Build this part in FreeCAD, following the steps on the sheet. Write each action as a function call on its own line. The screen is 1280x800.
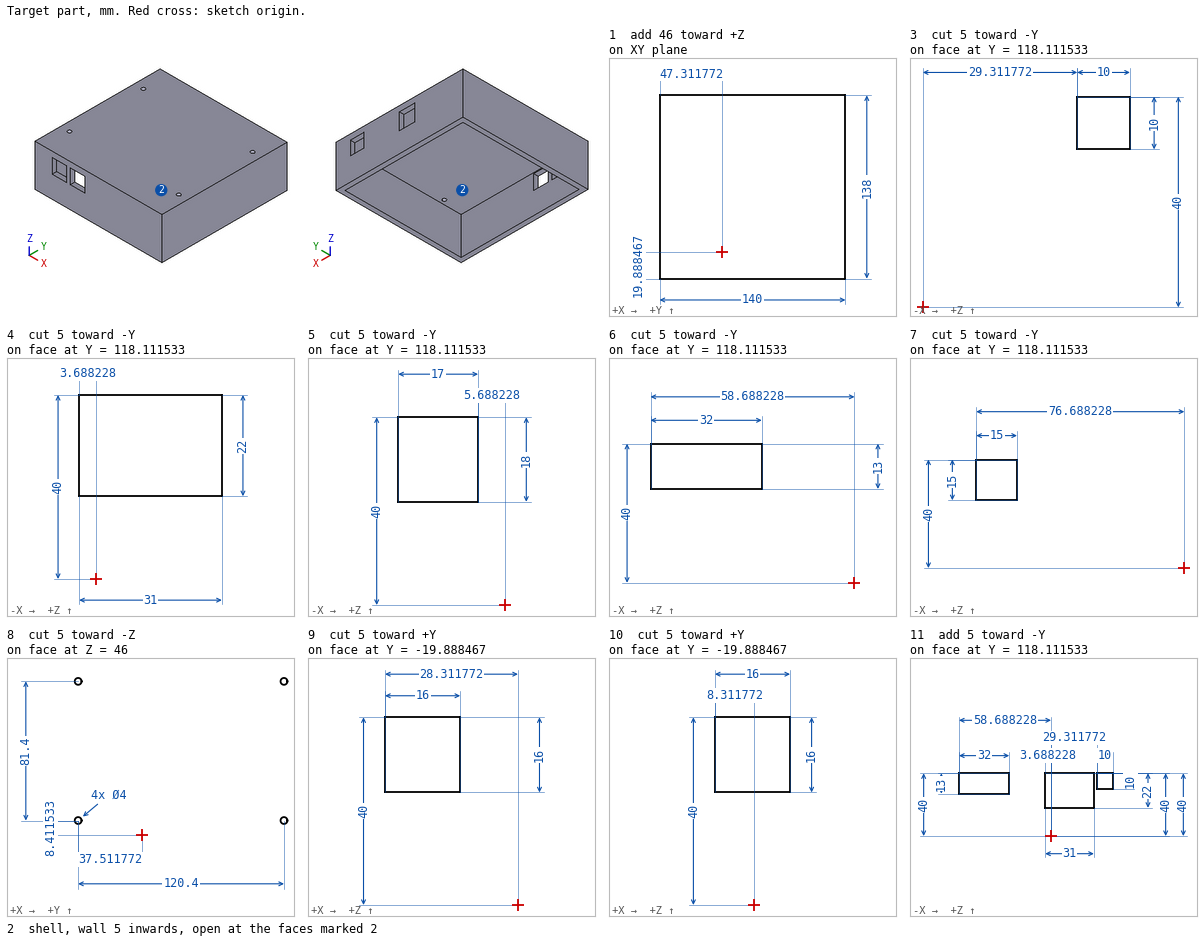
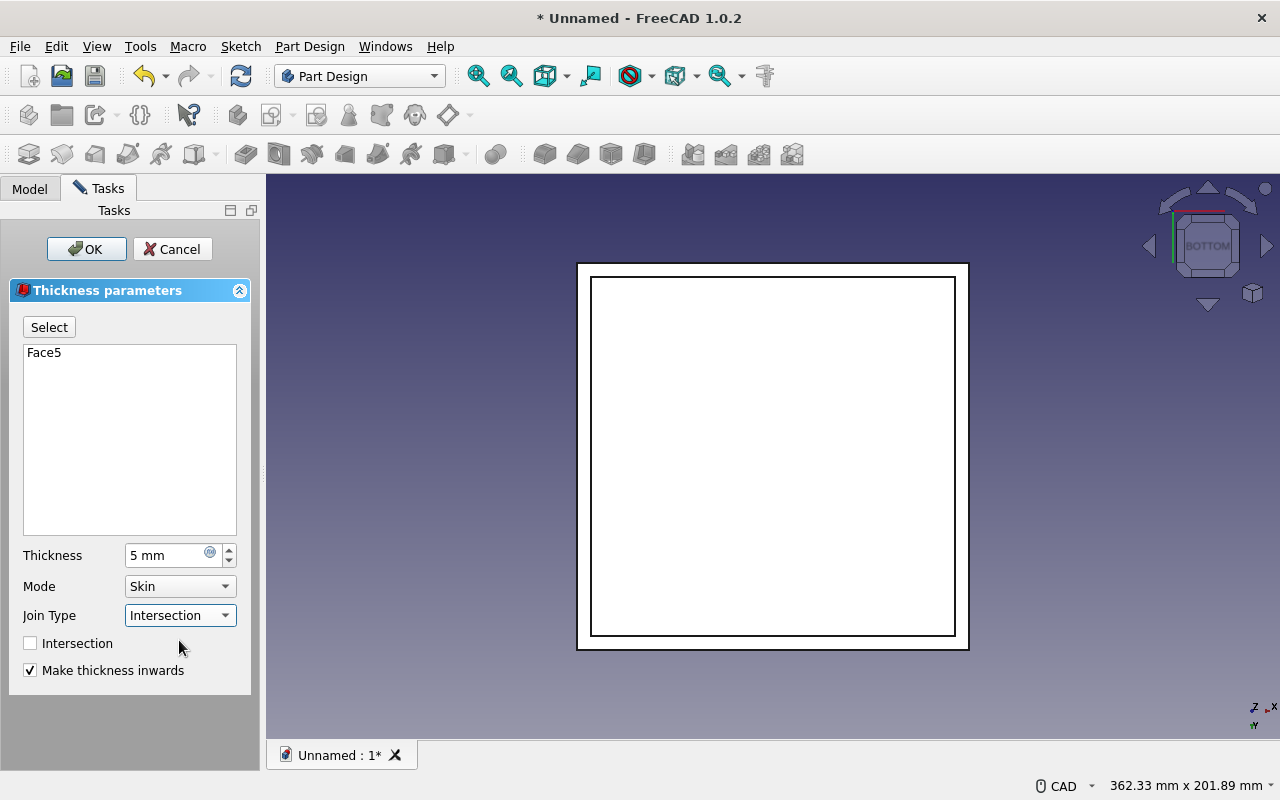
click(87, 249)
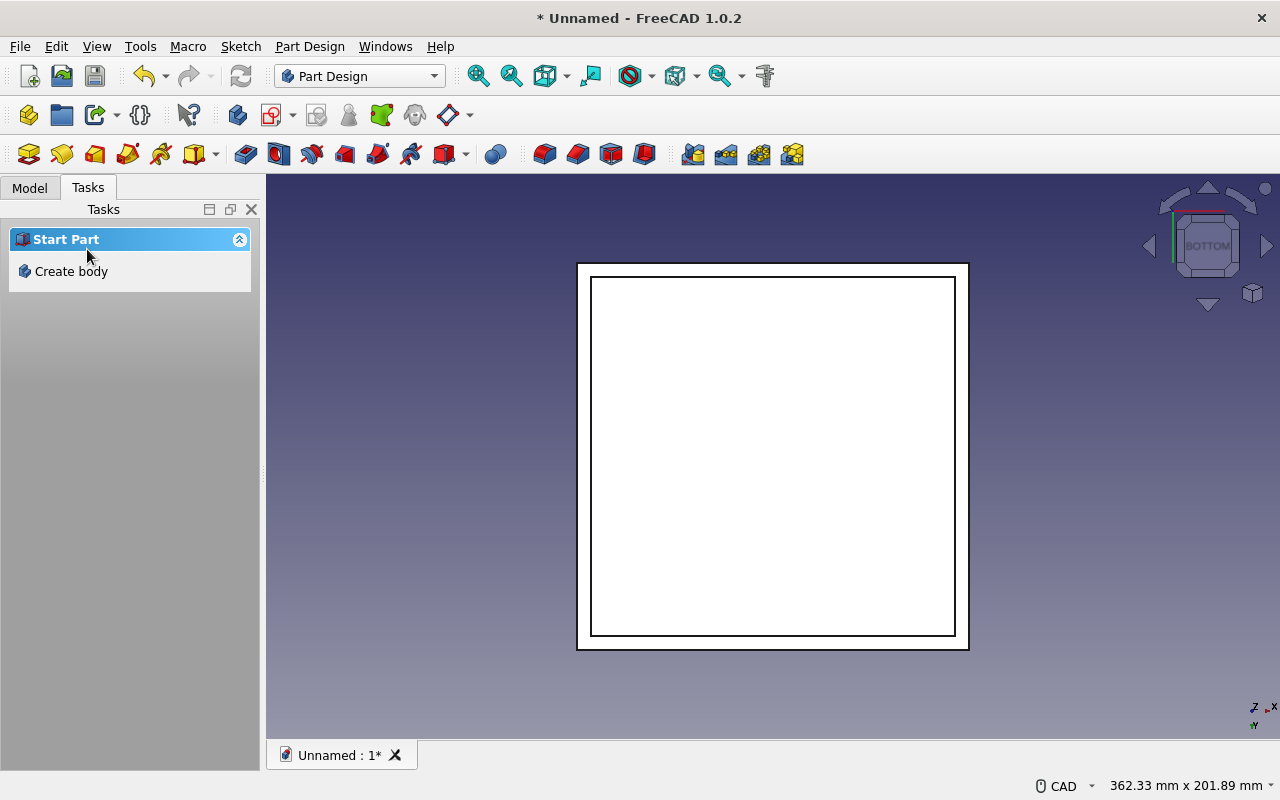
key(4)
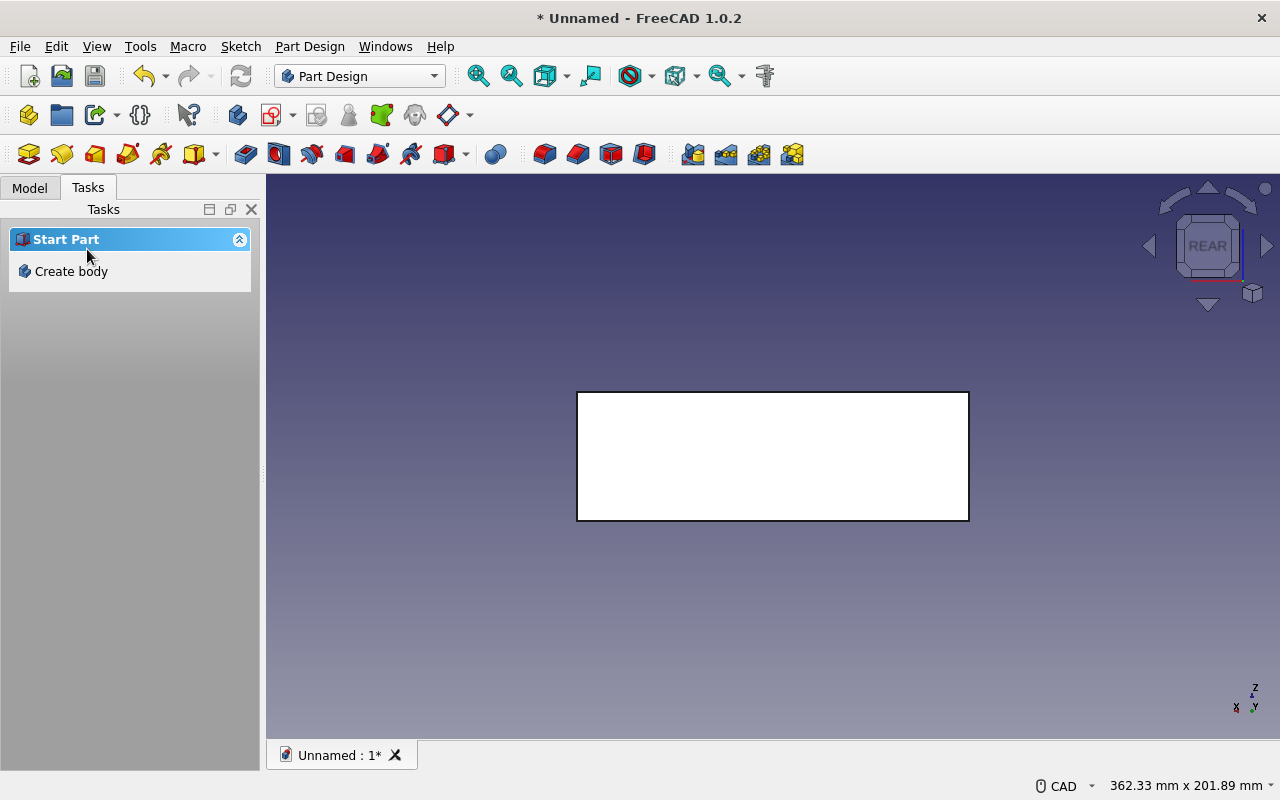
click(479, 76)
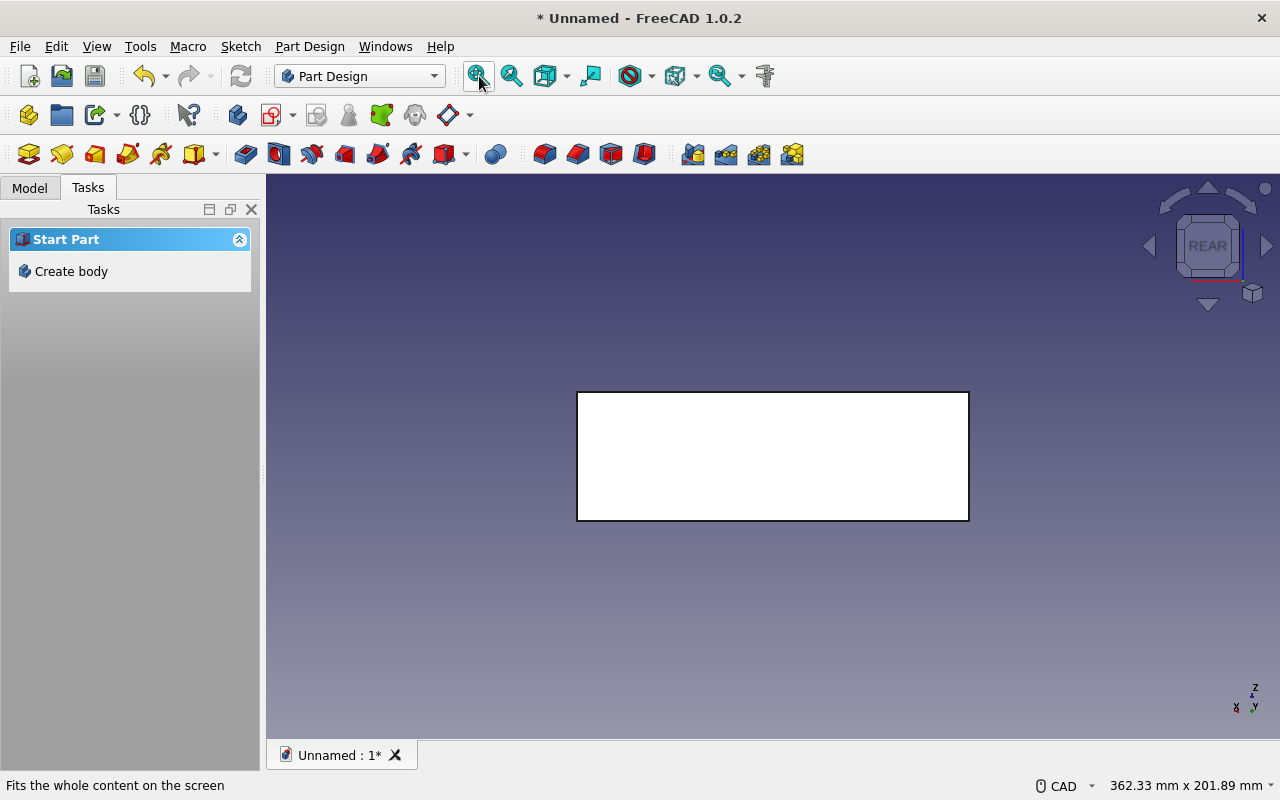
click(661, 456)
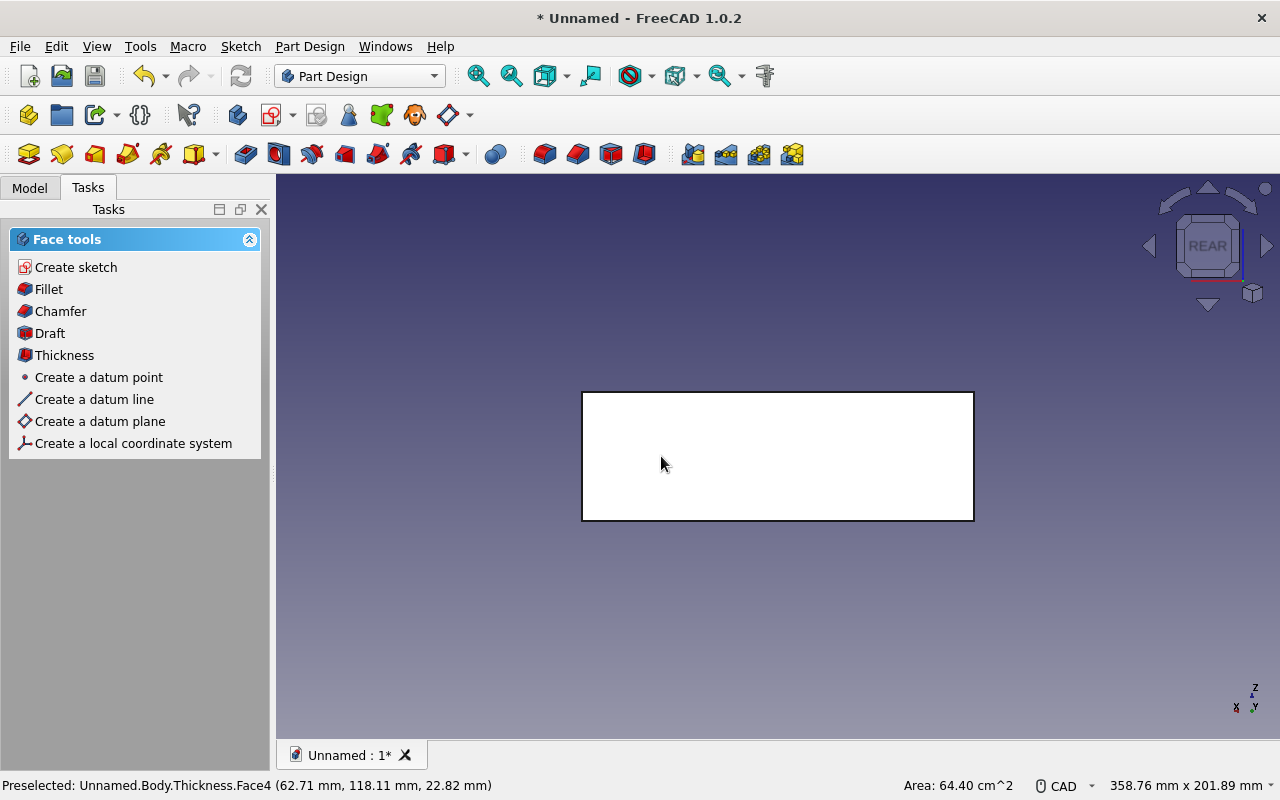
click(270, 116)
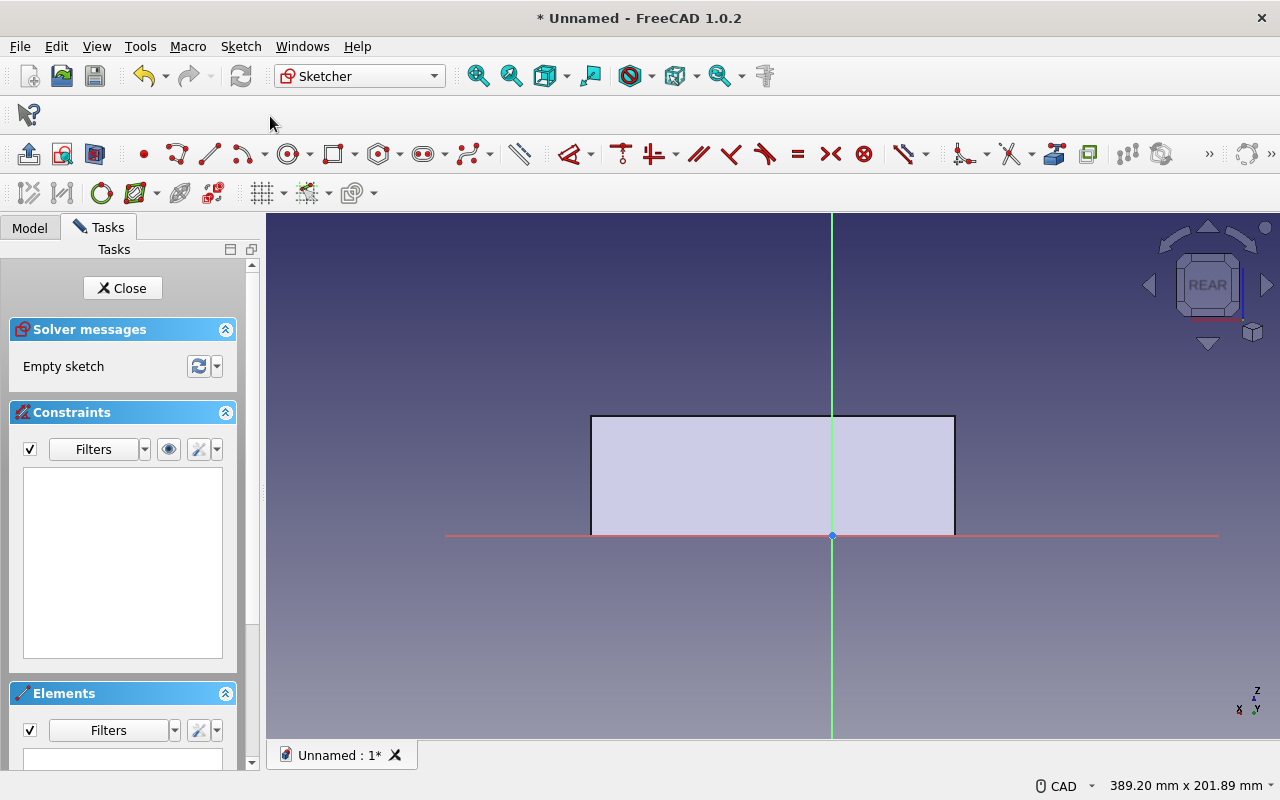
scroll(939, 442, up, 13)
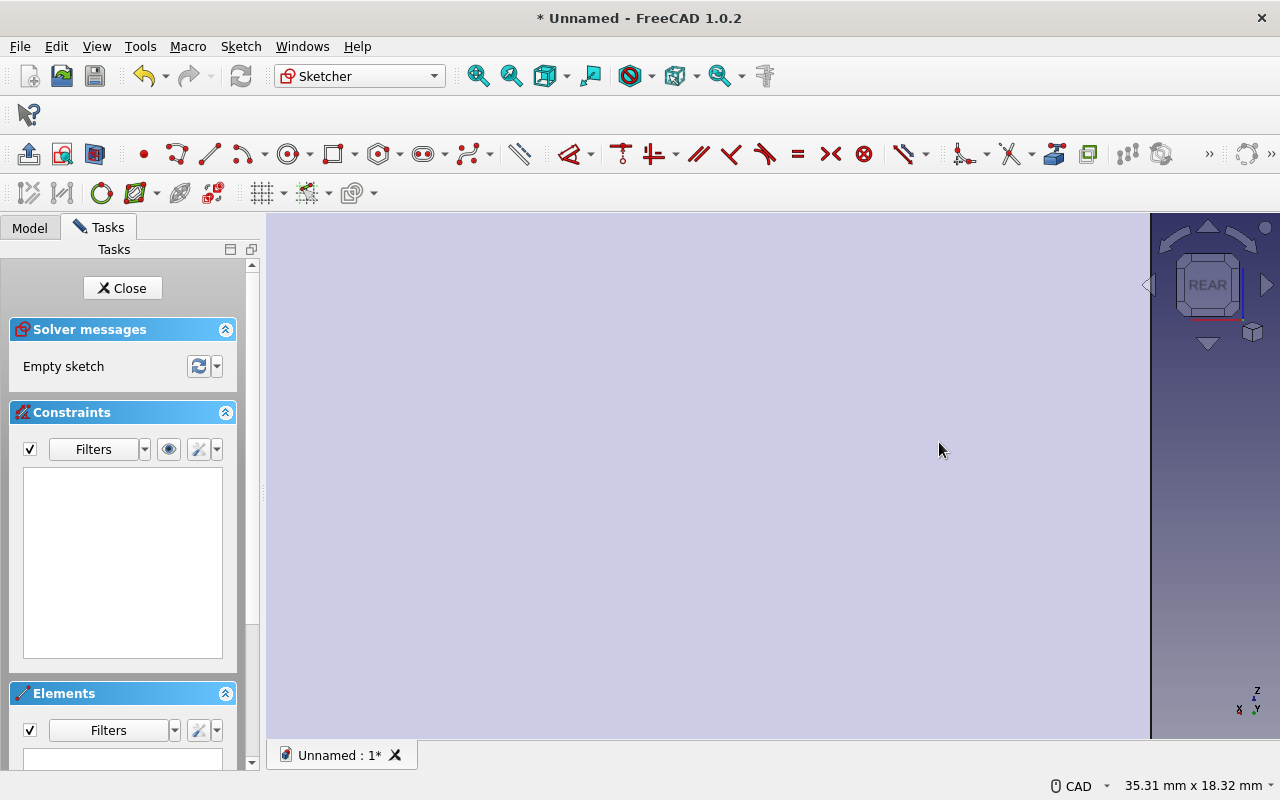
key(g)
key(r)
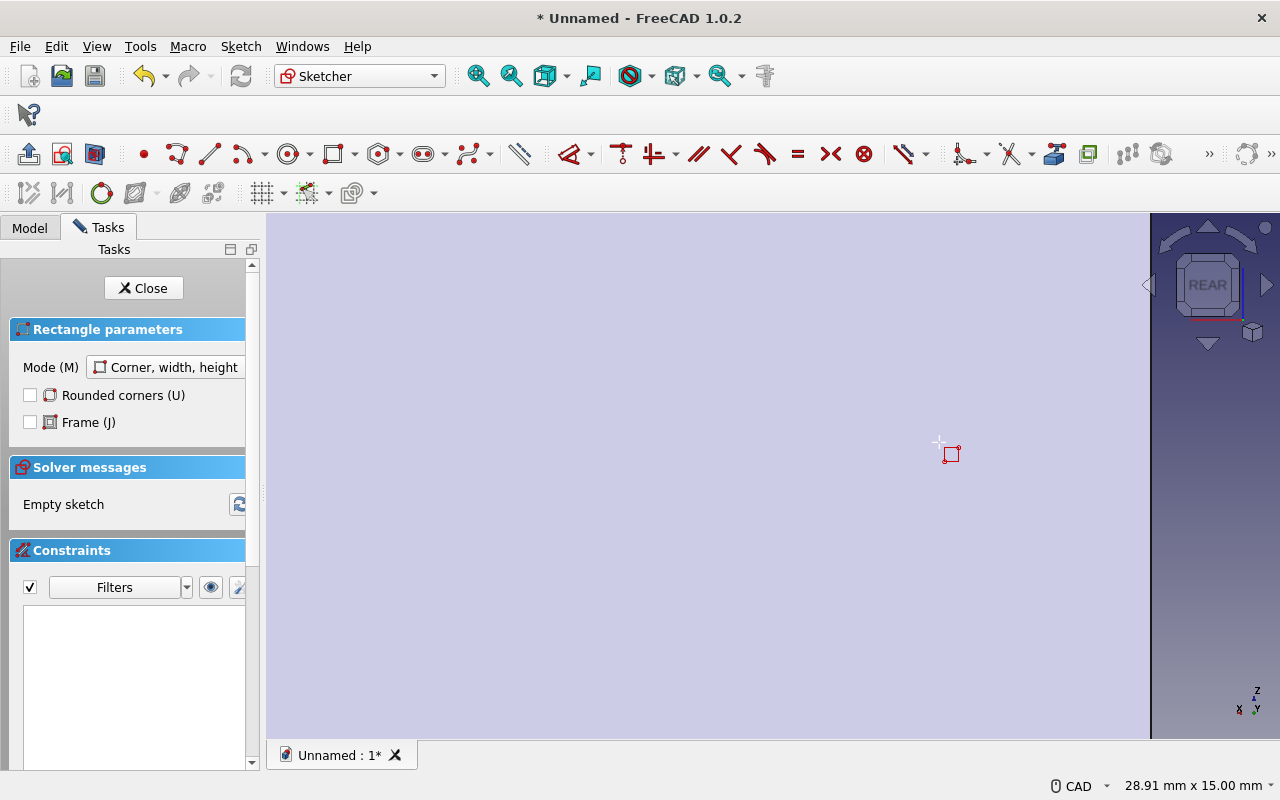
click(520, 298)
move(871, 649)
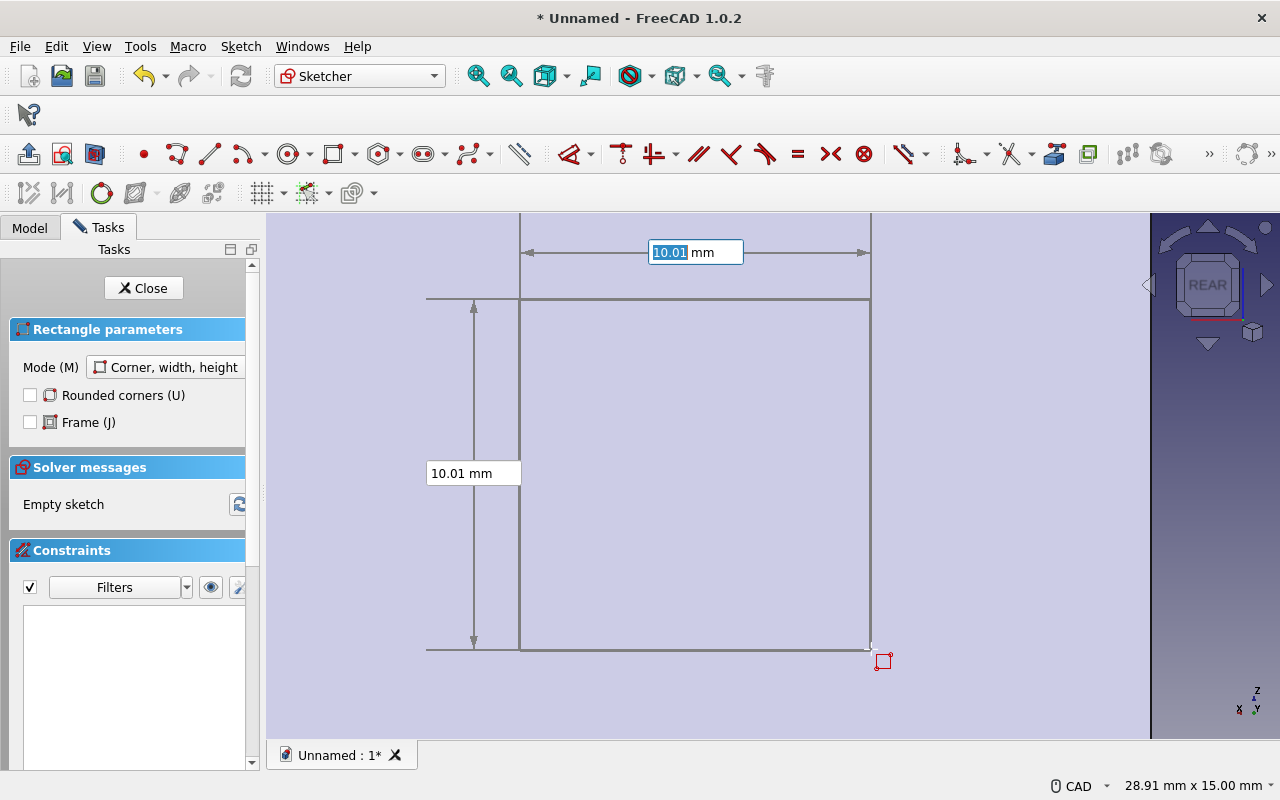
text(10)
key(Tab)
text(10)
key(Return)
key(Escape)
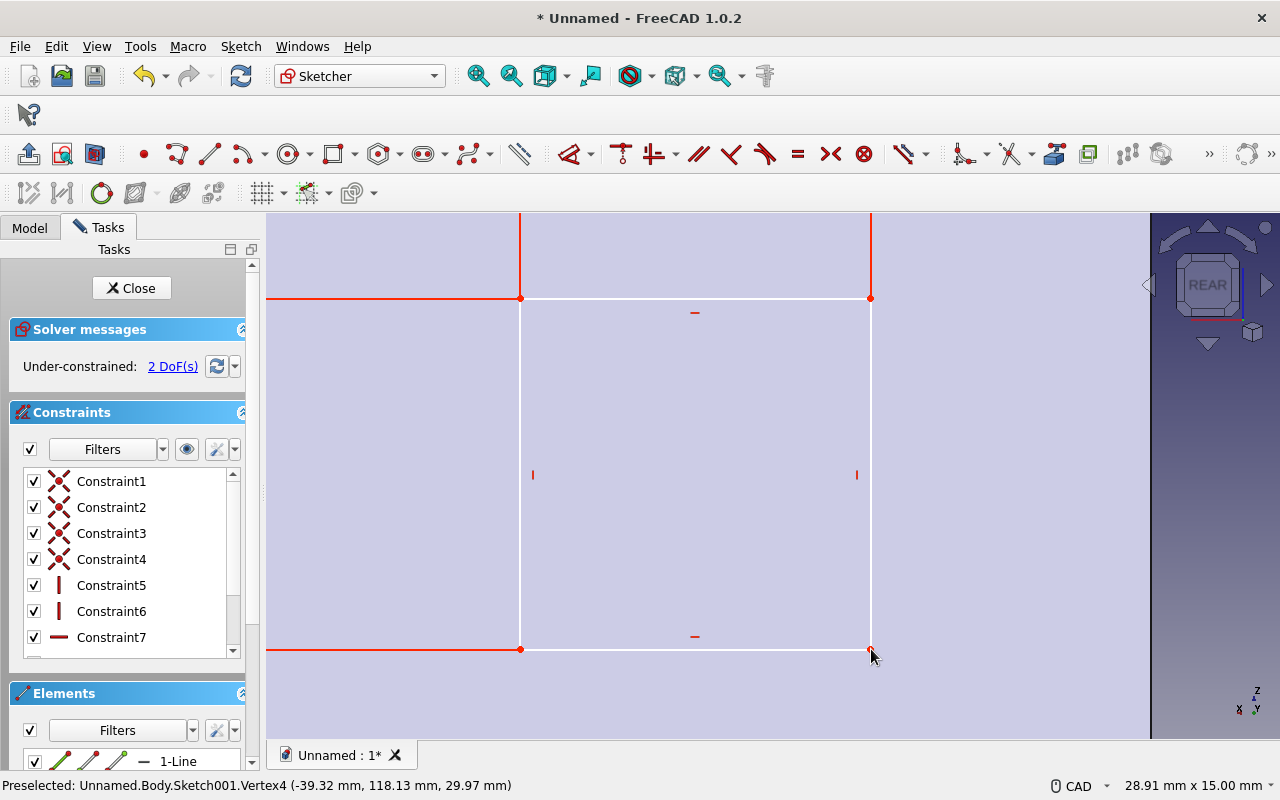
key(d)